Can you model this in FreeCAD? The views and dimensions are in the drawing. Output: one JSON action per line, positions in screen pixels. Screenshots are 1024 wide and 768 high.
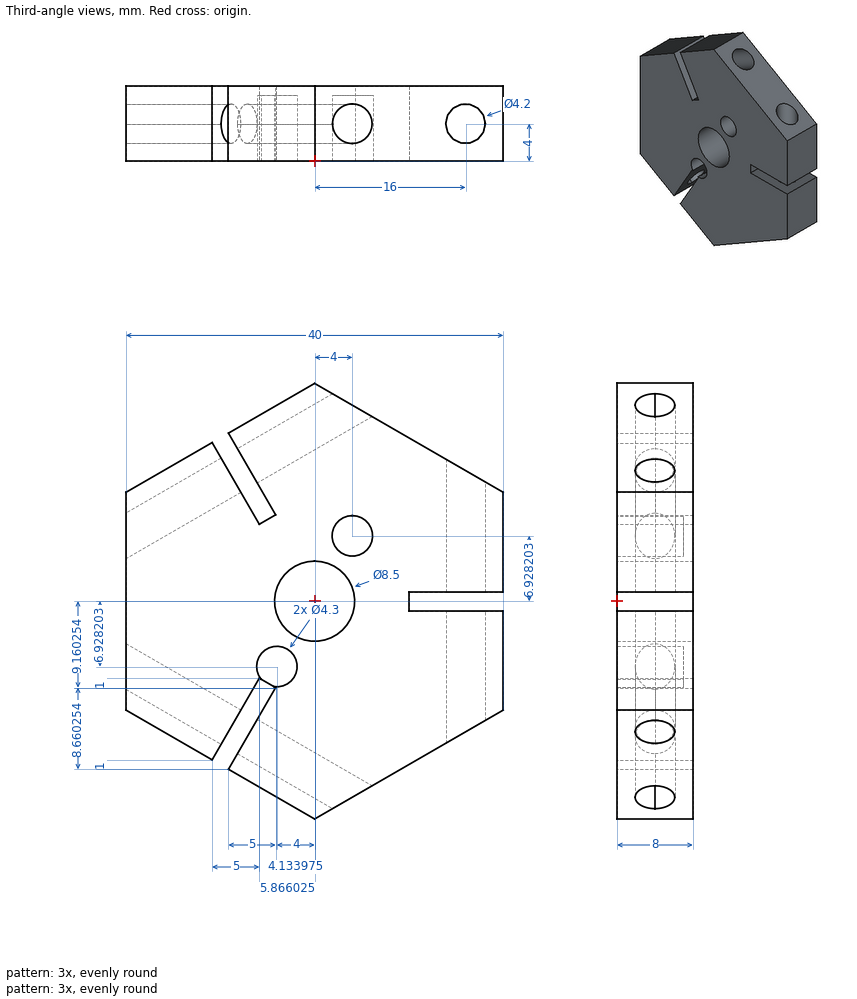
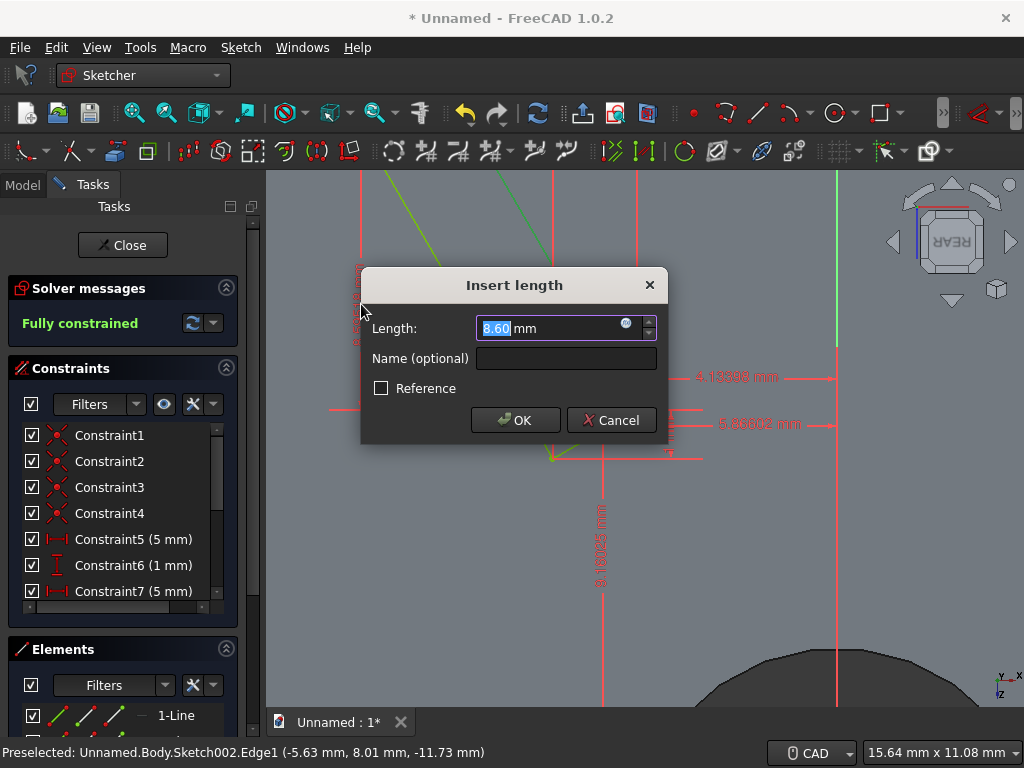
{"action": "type", "text": "8.660254"}
{"action": "key", "text": "Return"}
{"action": "key", "text": "Escape"}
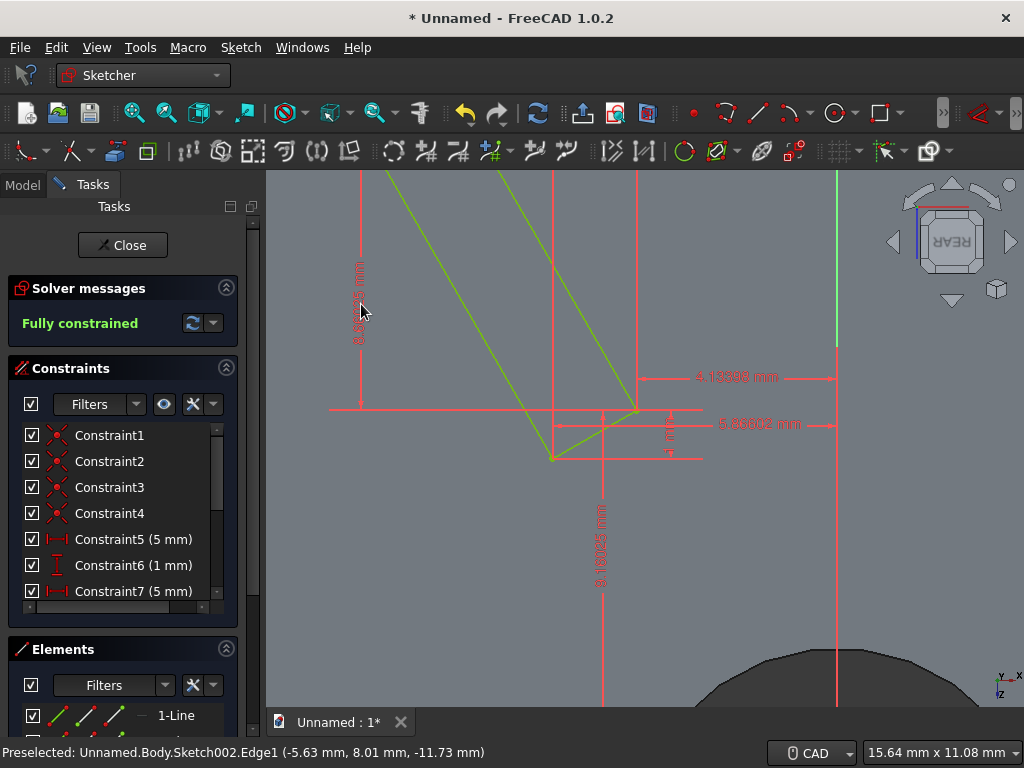
{"action": "left_click", "coordinate": [123, 245]}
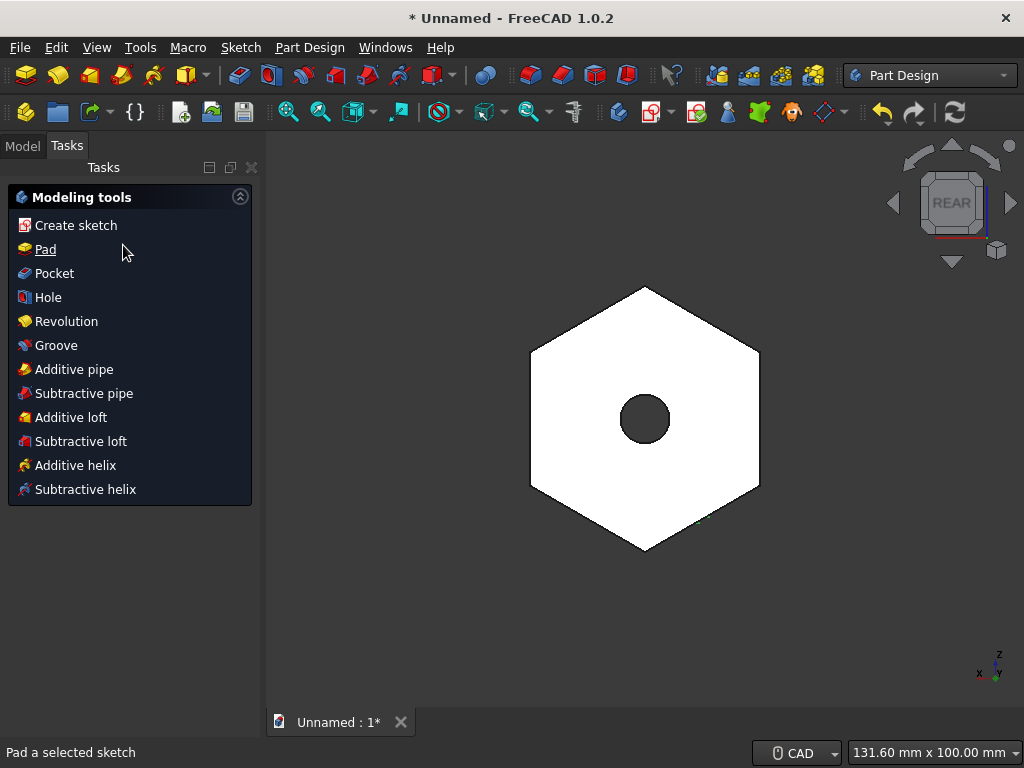
{"action": "left_click", "coordinate": [240, 76]}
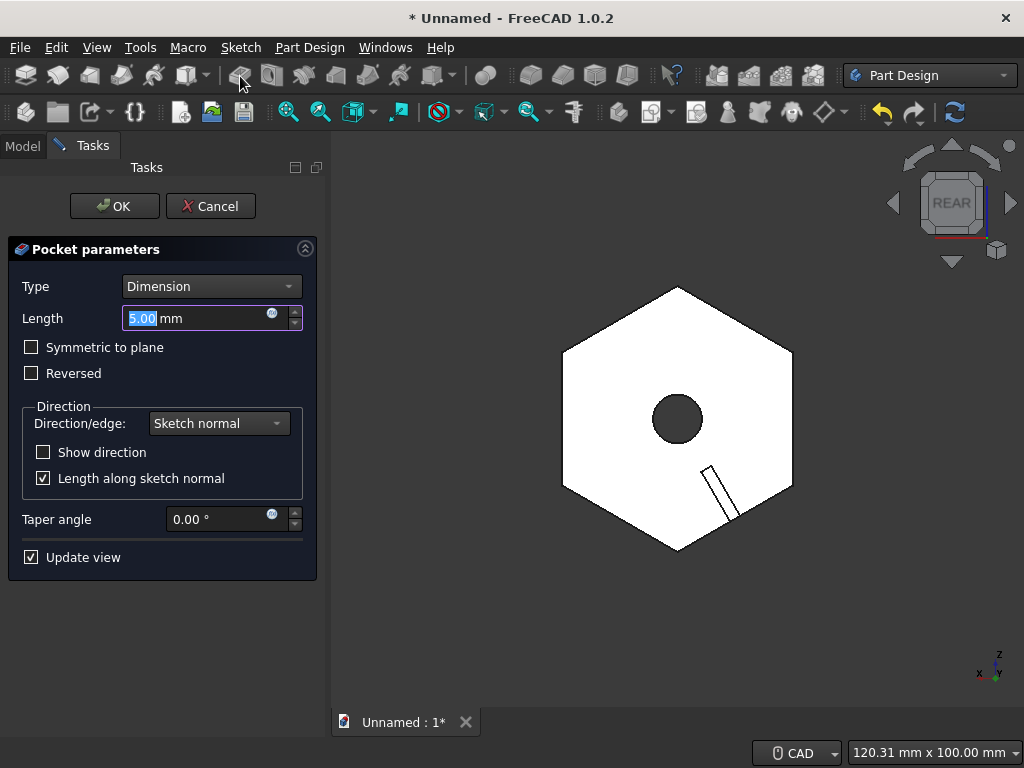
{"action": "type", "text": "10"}
{"action": "key", "text": "Tab"}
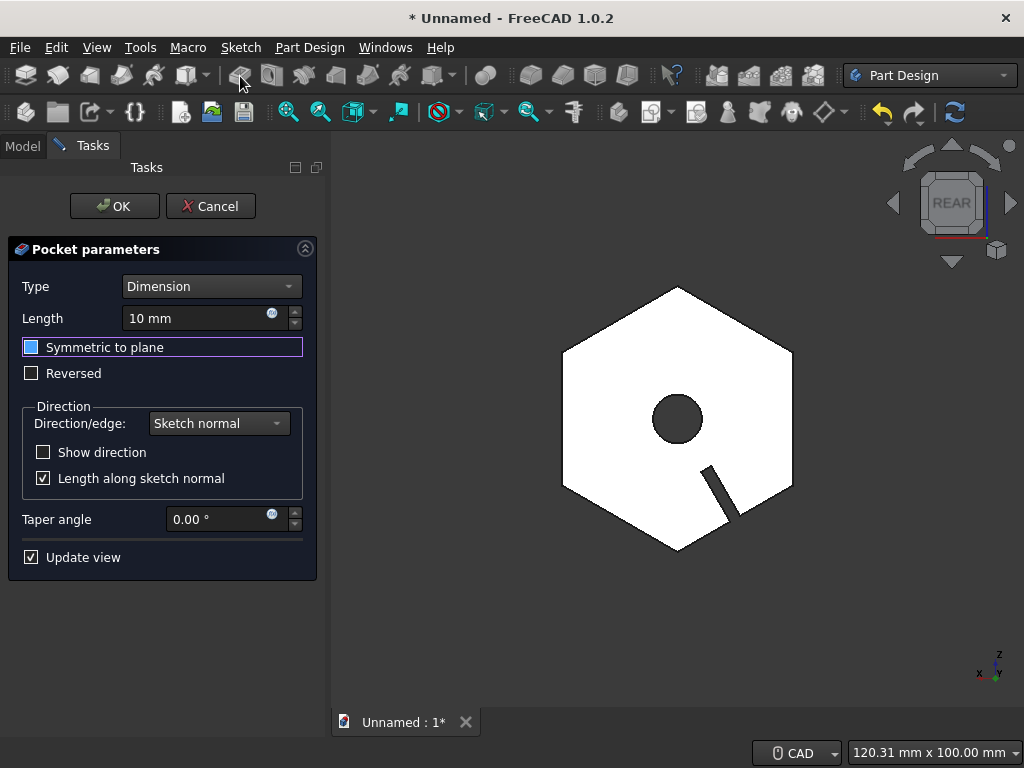
{"action": "left_click", "coordinate": [115, 206]}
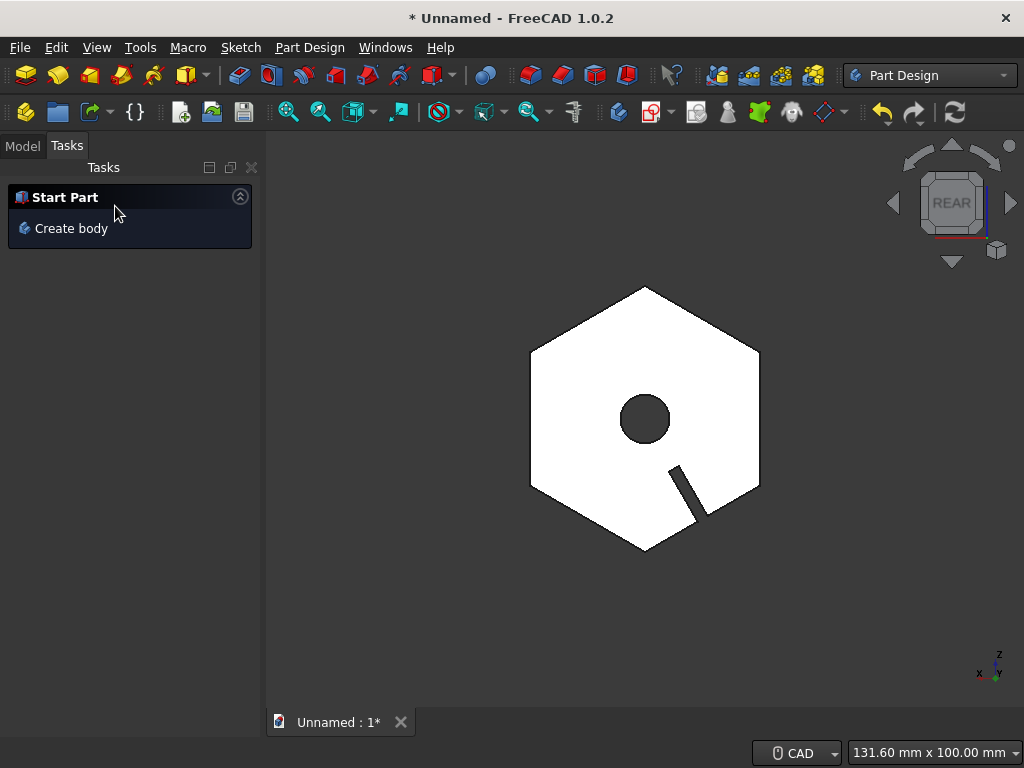
{"action": "left_click", "coordinate": [23, 145]}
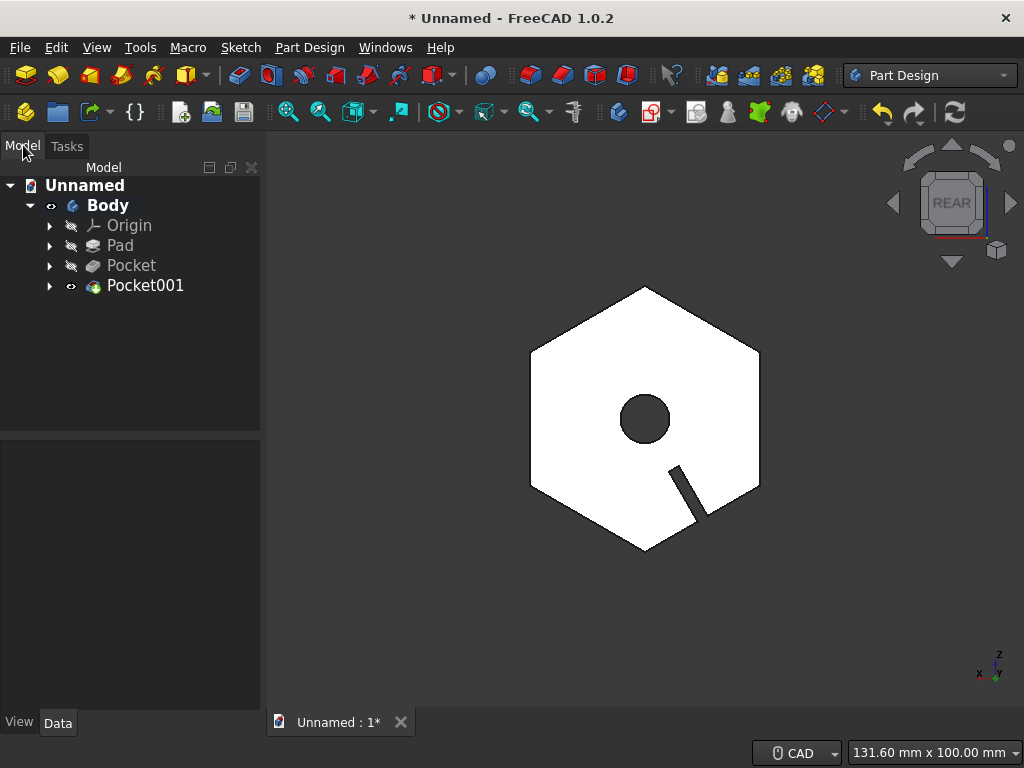
{"action": "left_click", "coordinate": [116, 286]}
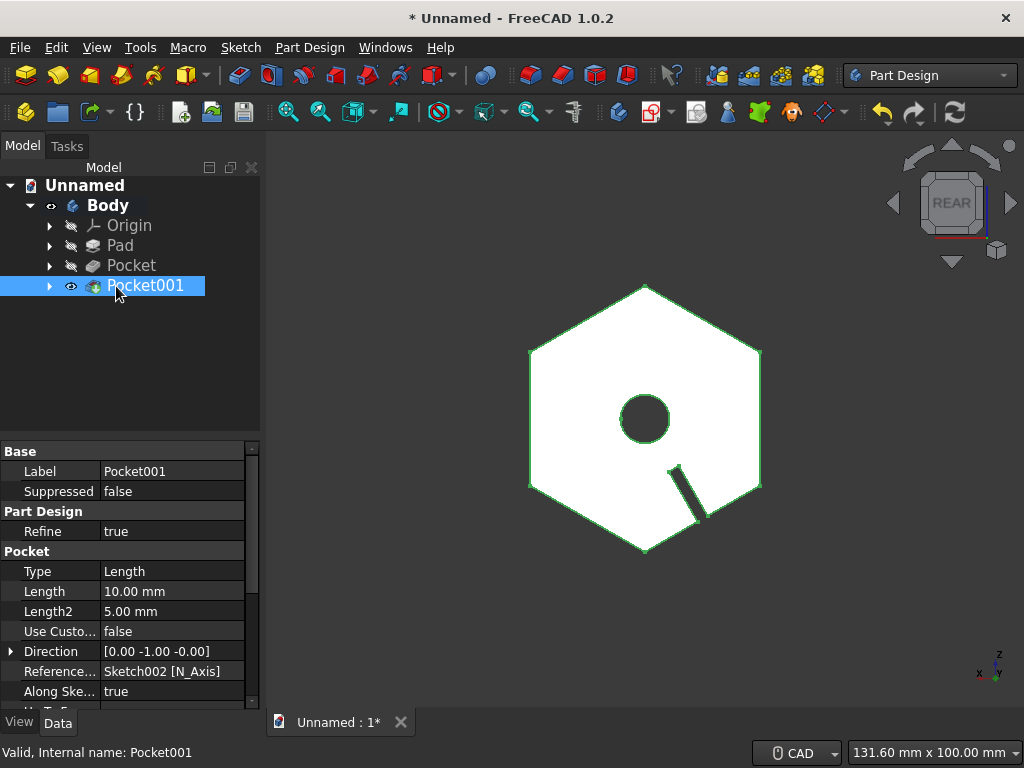
{"action": "left_click", "coordinate": [782, 76]}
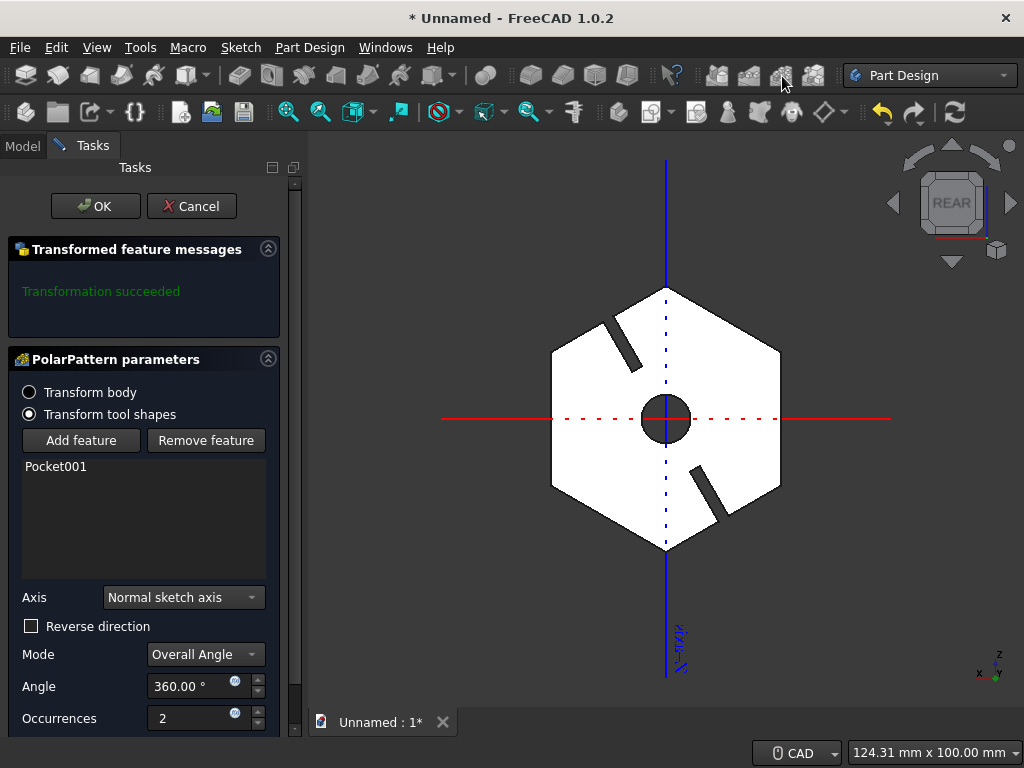
{"action": "left_click", "coordinate": [184, 598]}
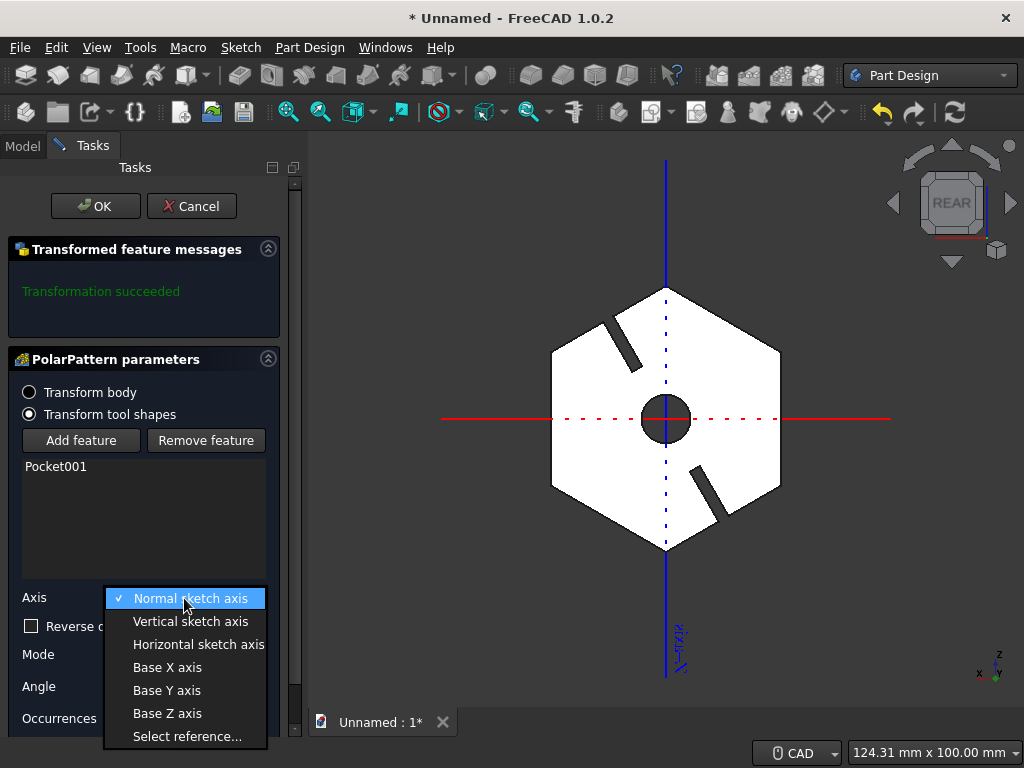
{"action": "left_click", "coordinate": [184, 690]}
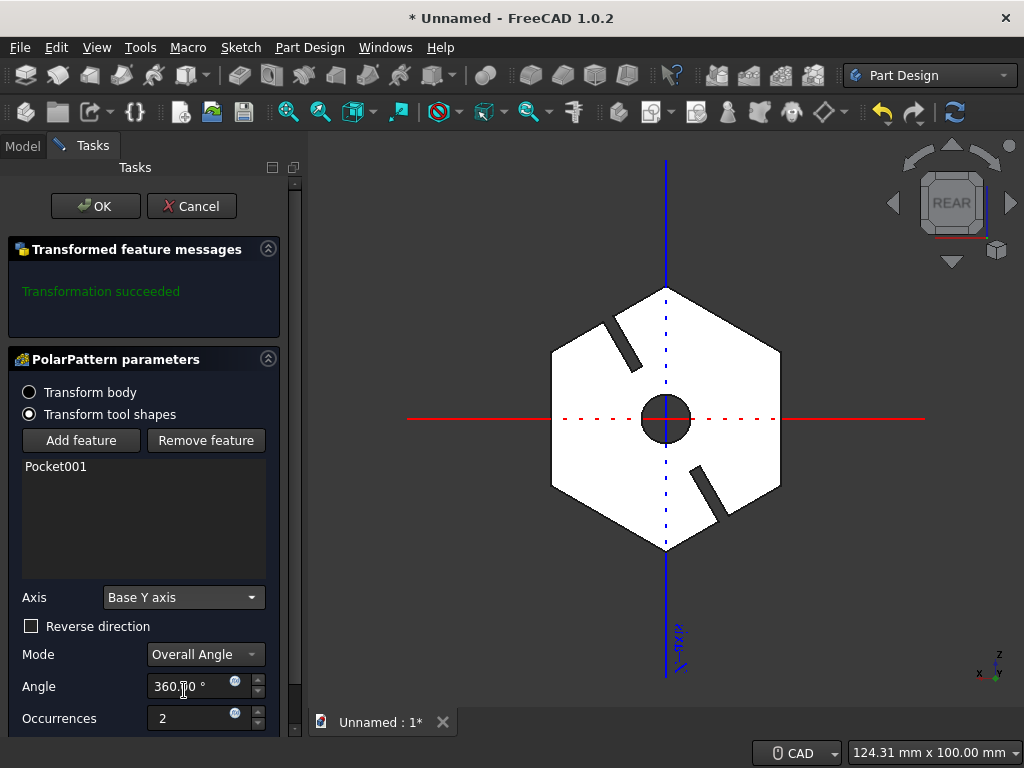
{"action": "triple_click", "coordinate": [198, 718]}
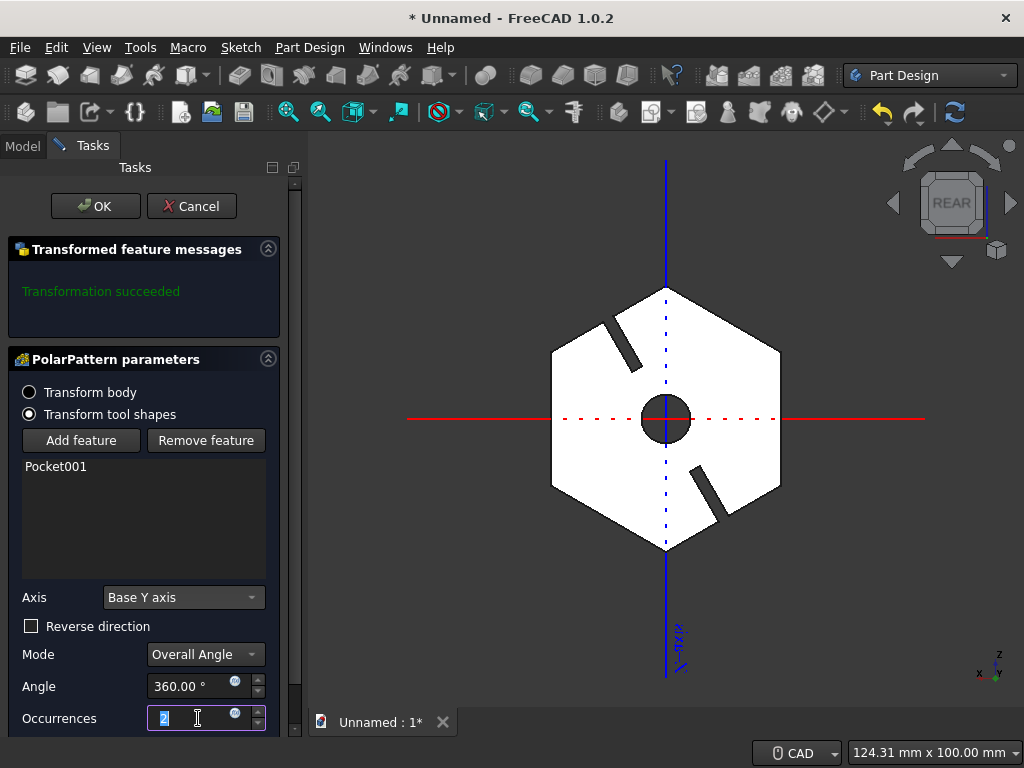
{"action": "type", "text": "3"}
{"action": "key", "text": "Tab"}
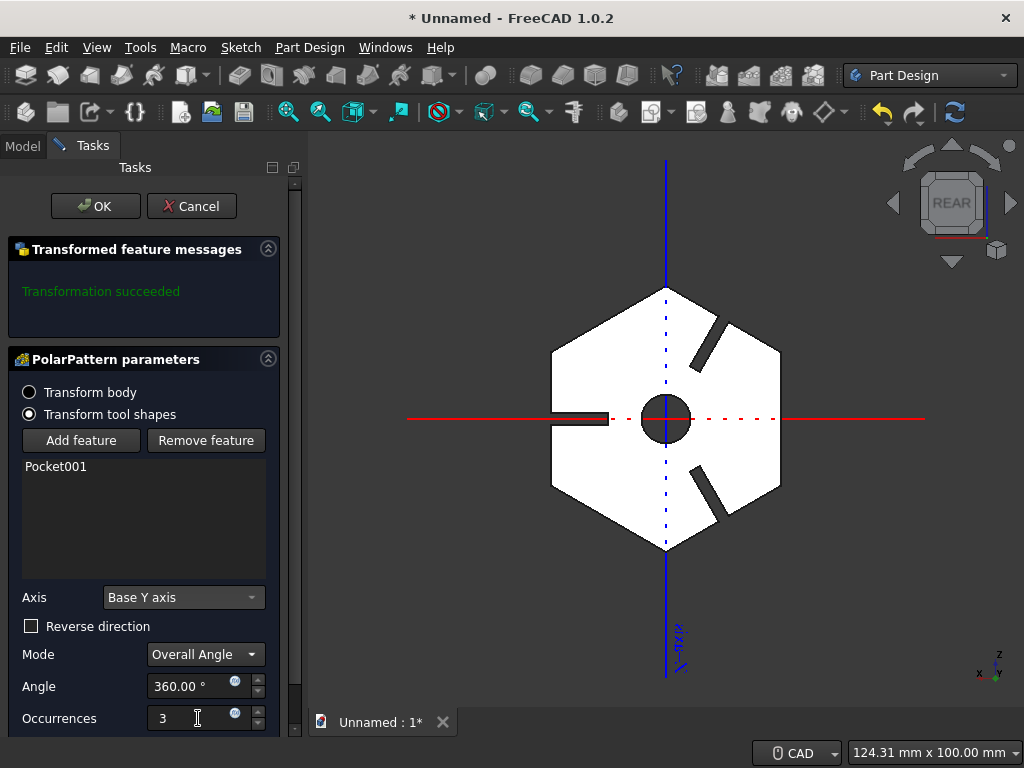
{"action": "left_click", "coordinate": [96, 206]}